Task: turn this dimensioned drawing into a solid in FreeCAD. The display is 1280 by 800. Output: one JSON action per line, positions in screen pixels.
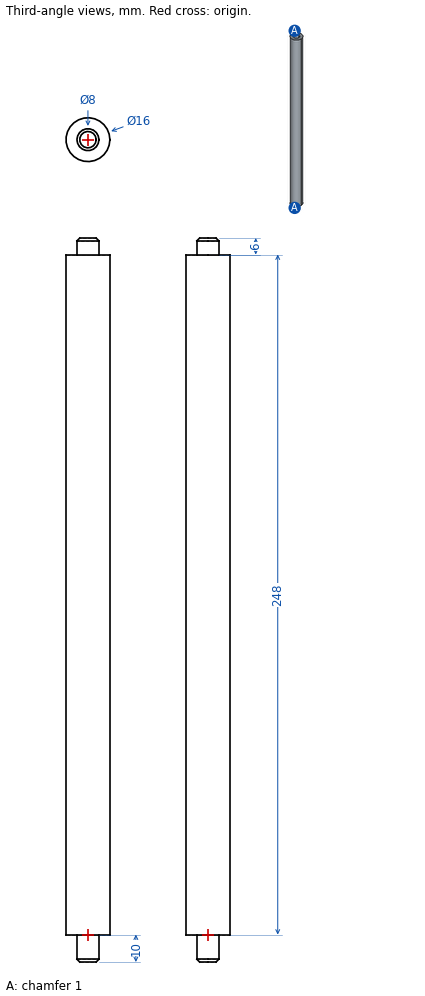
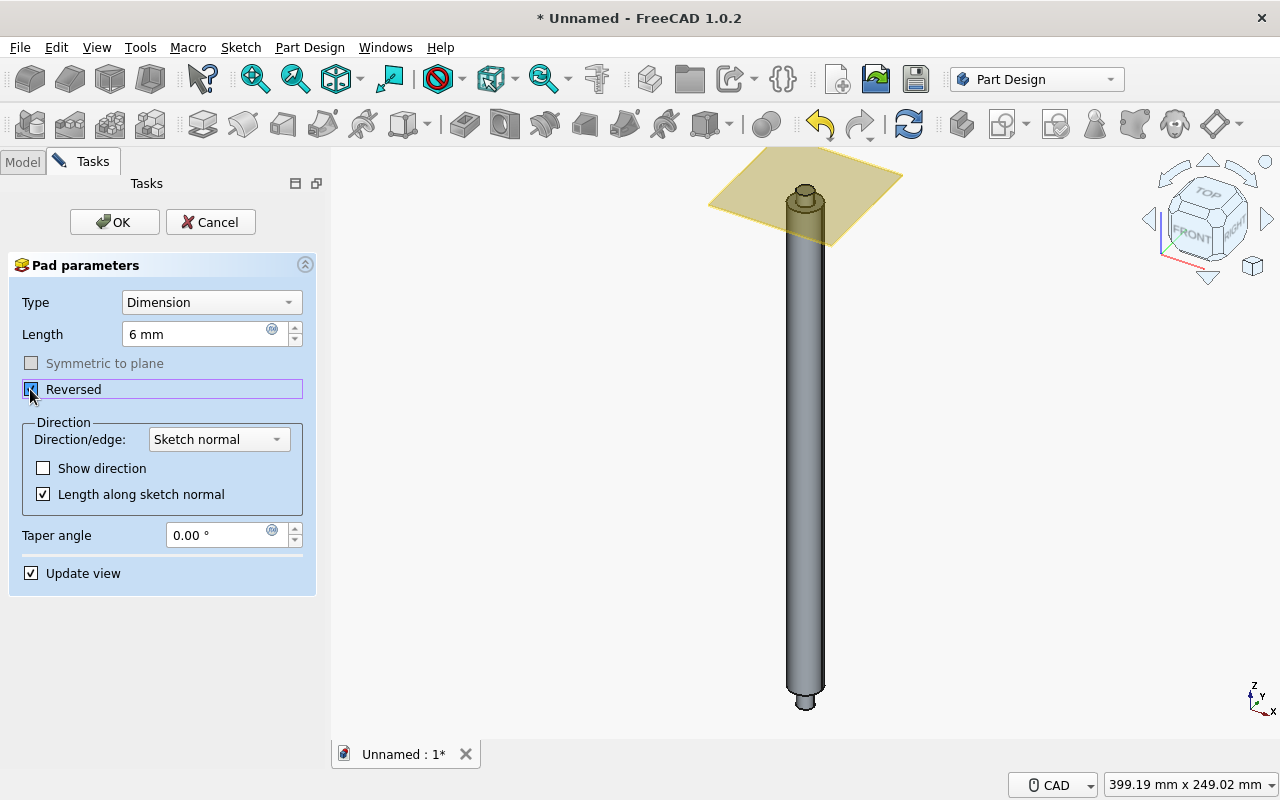
{"action": "left_click", "coordinate": [115, 222]}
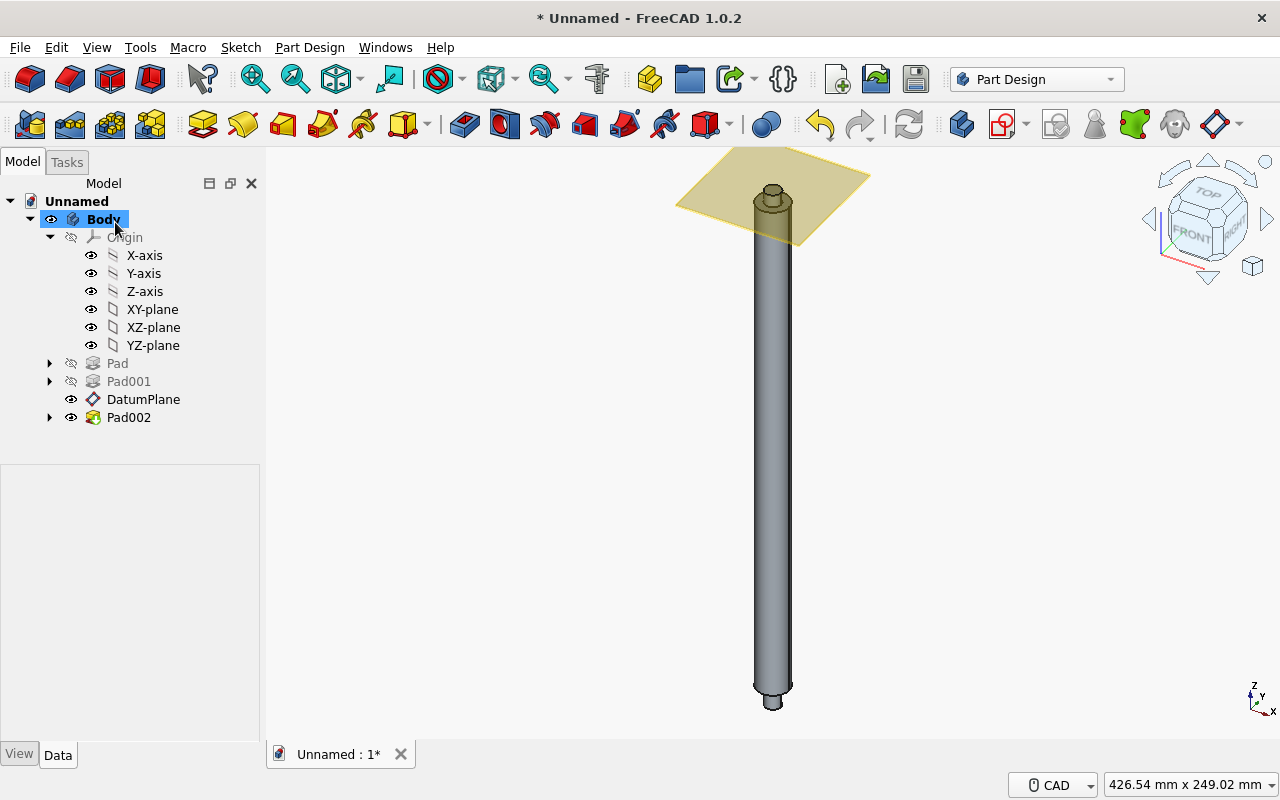
{"action": "left_click", "coordinate": [116, 399]}
{"action": "key", "text": "space"}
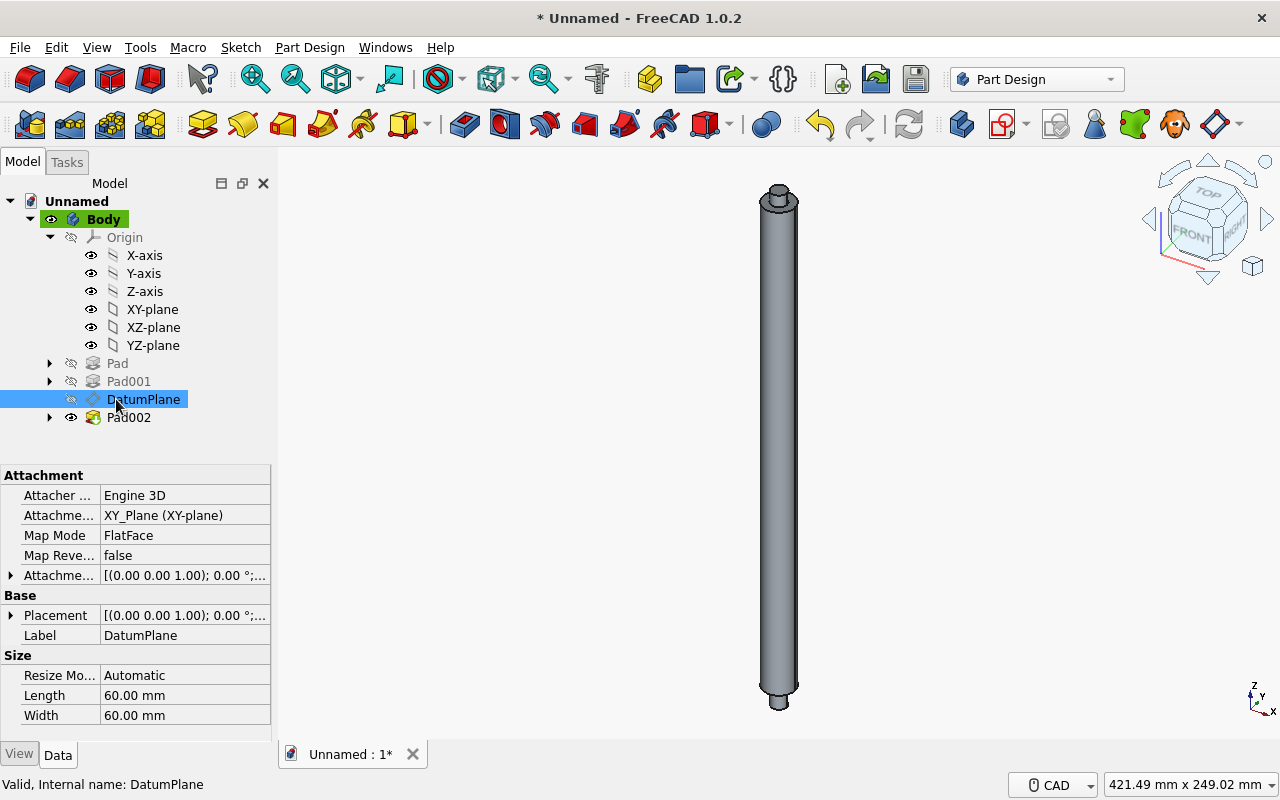
{"action": "left_click", "coordinate": [771, 187]}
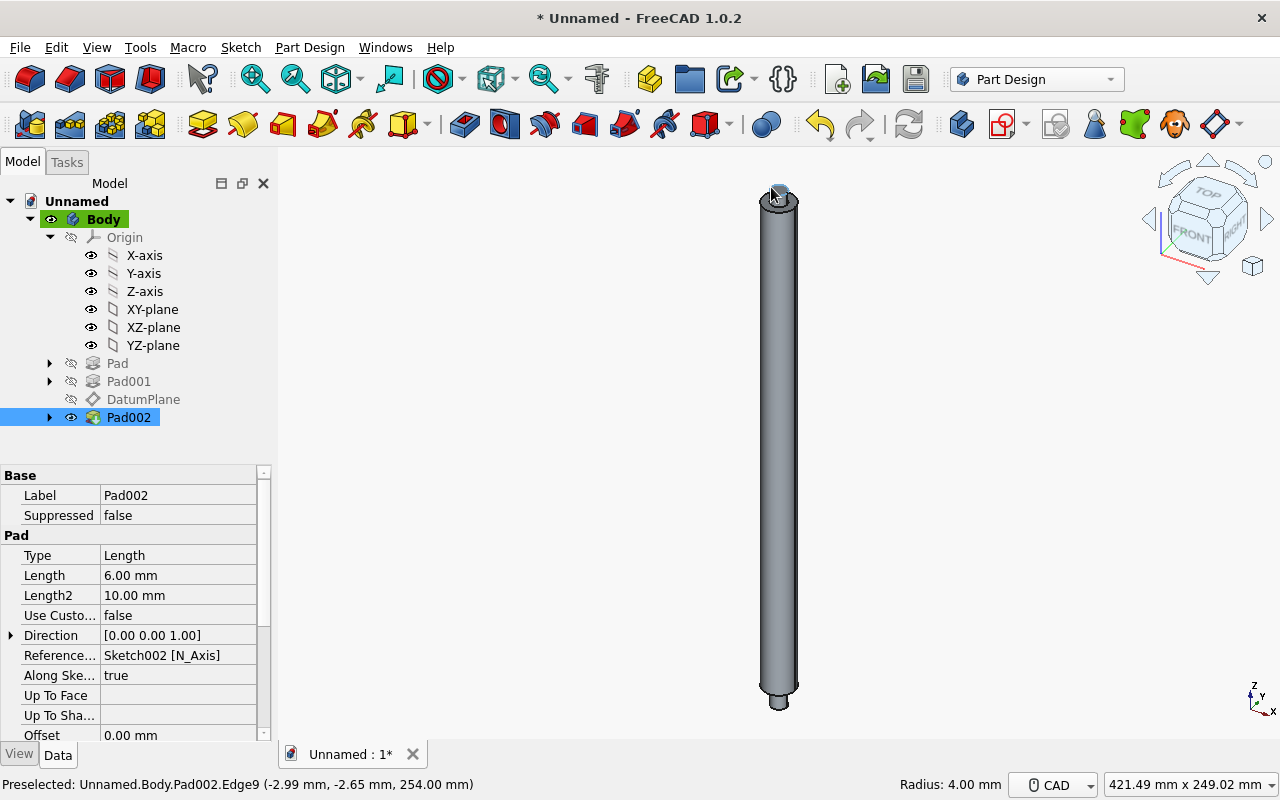
{"action": "left_click", "coordinate": [772, 707], "text": "ctrl"}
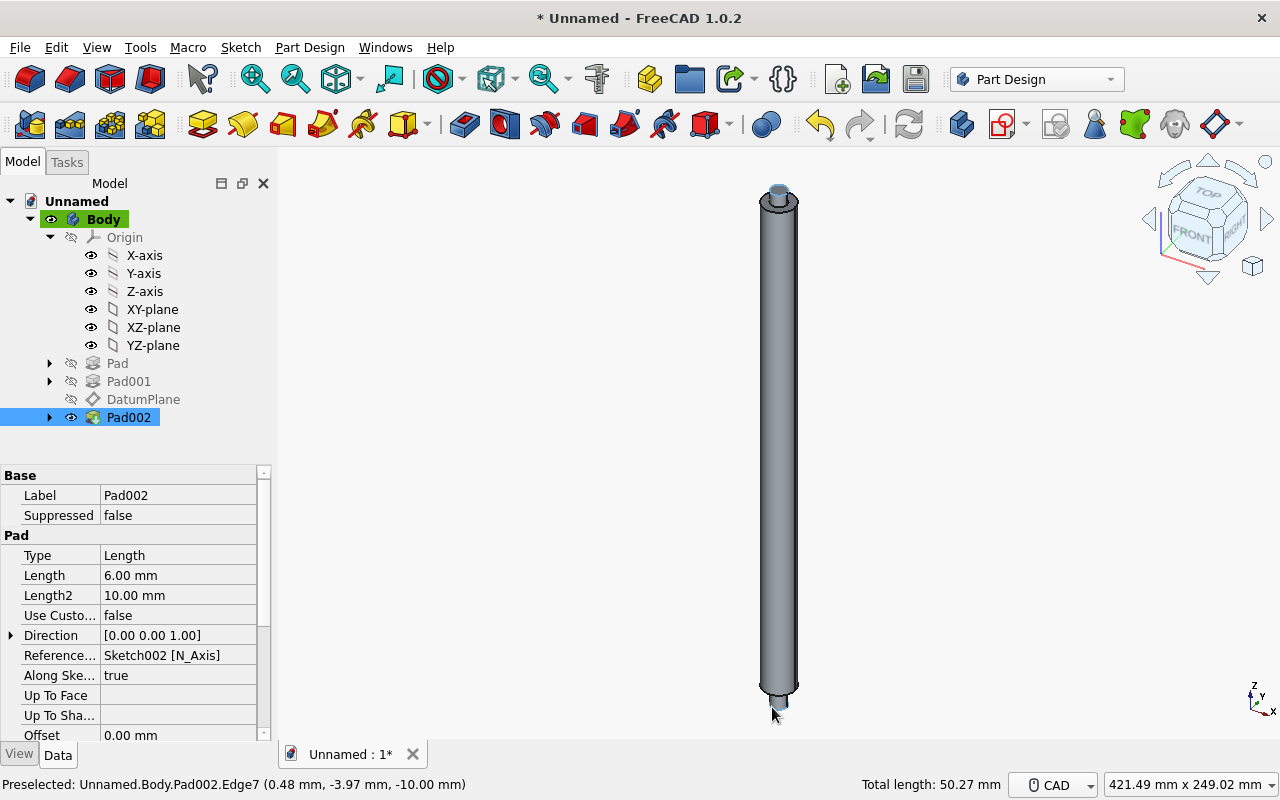
{"action": "left_click", "coordinate": [70, 80]}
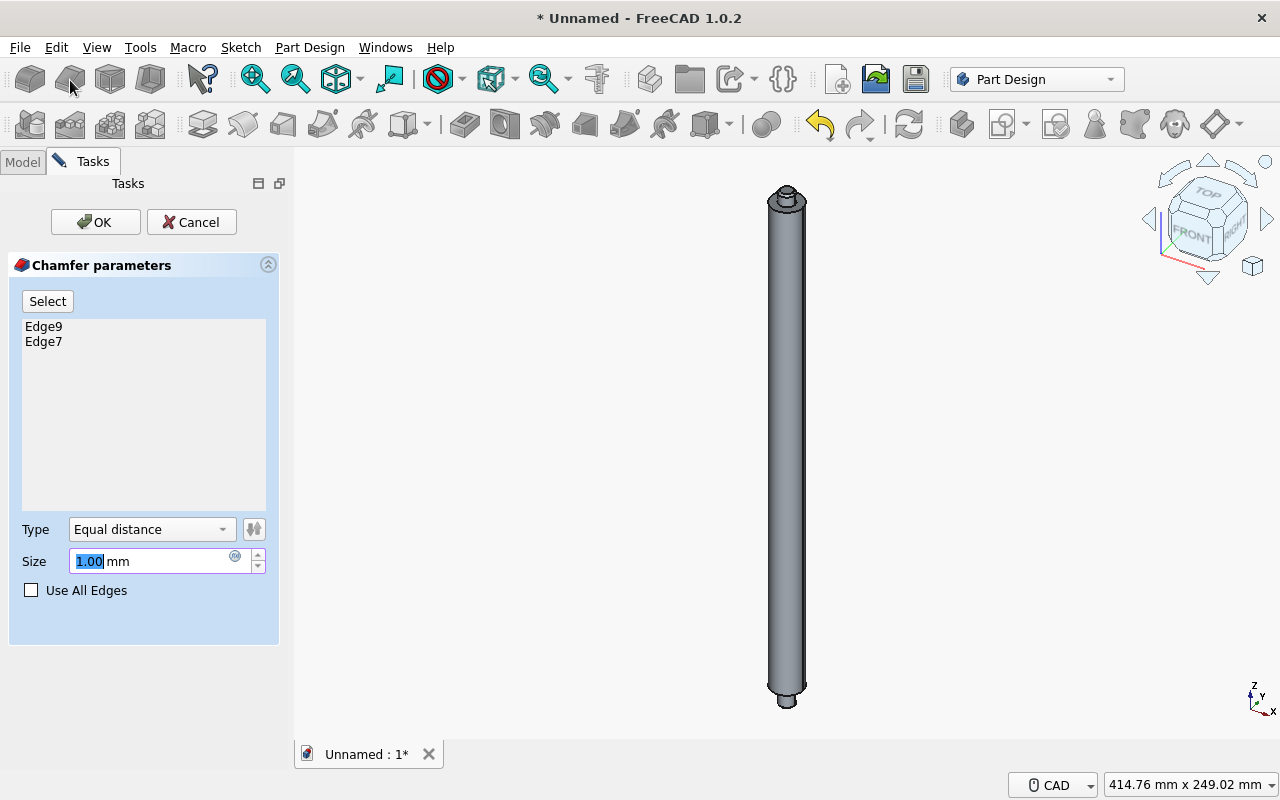
{"action": "type", "text": "1"}
{"action": "key", "text": "Tab"}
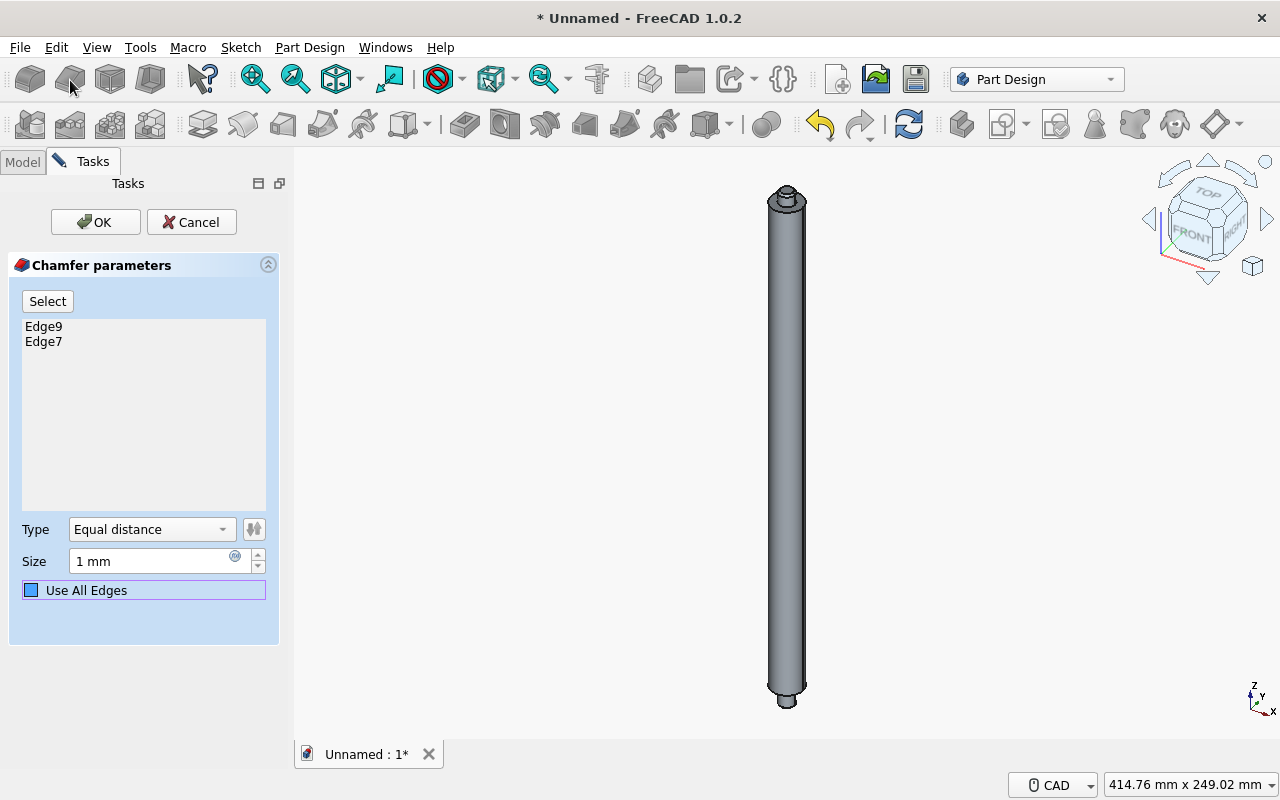
{"action": "left_click", "coordinate": [96, 222]}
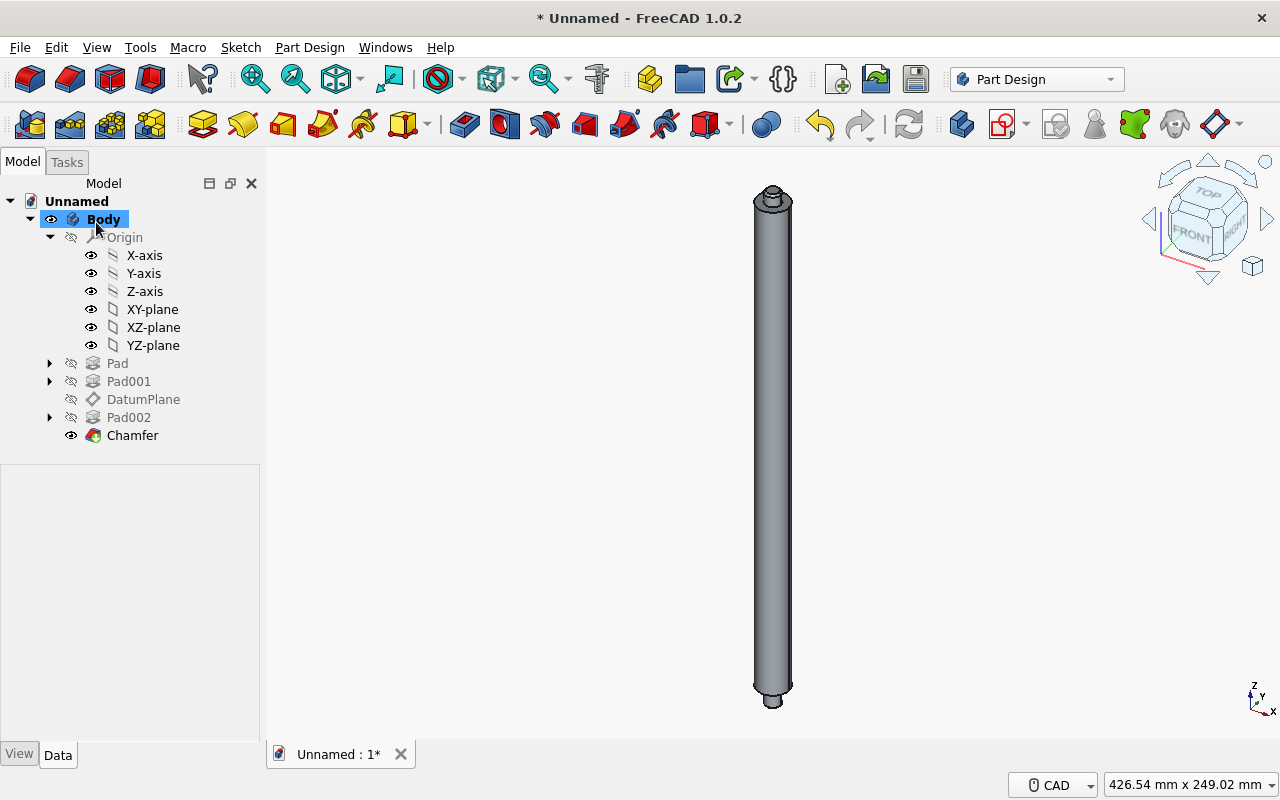
{"action": "key", "text": "0"}